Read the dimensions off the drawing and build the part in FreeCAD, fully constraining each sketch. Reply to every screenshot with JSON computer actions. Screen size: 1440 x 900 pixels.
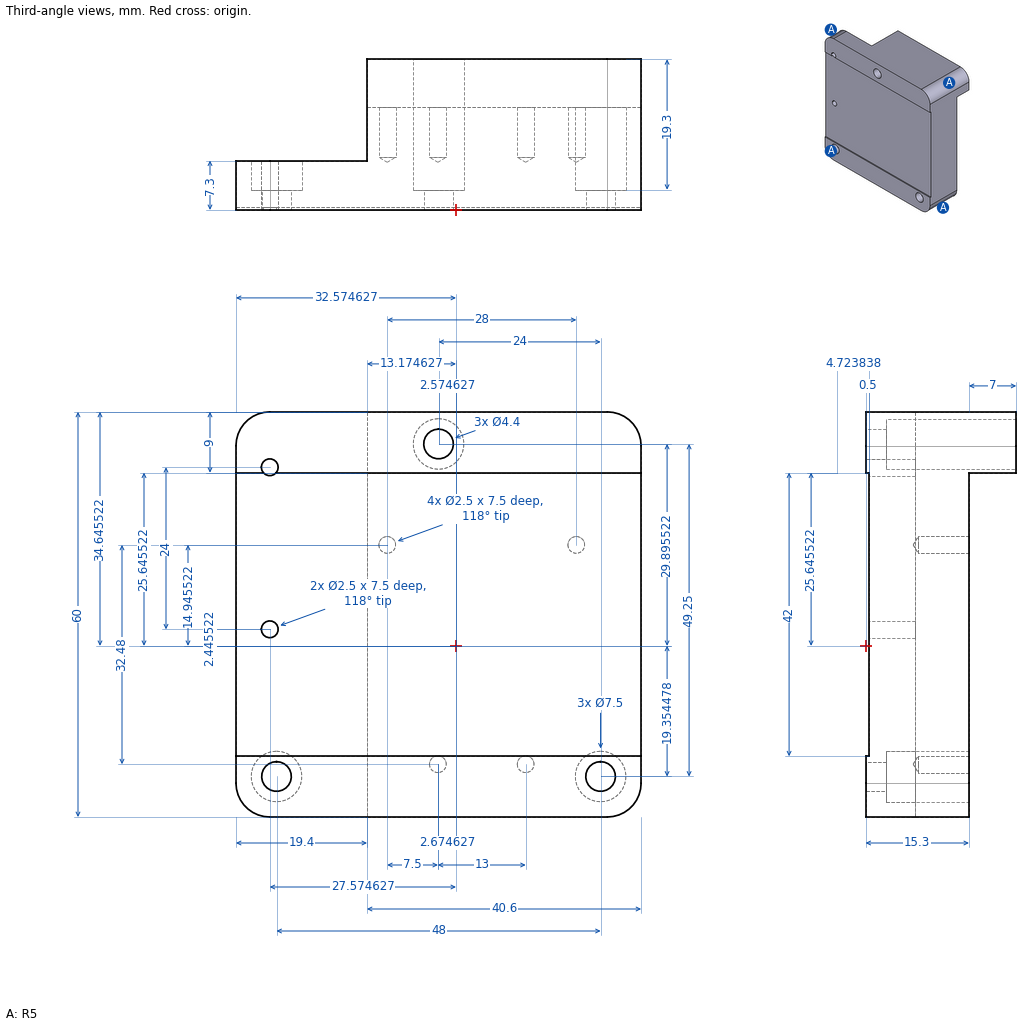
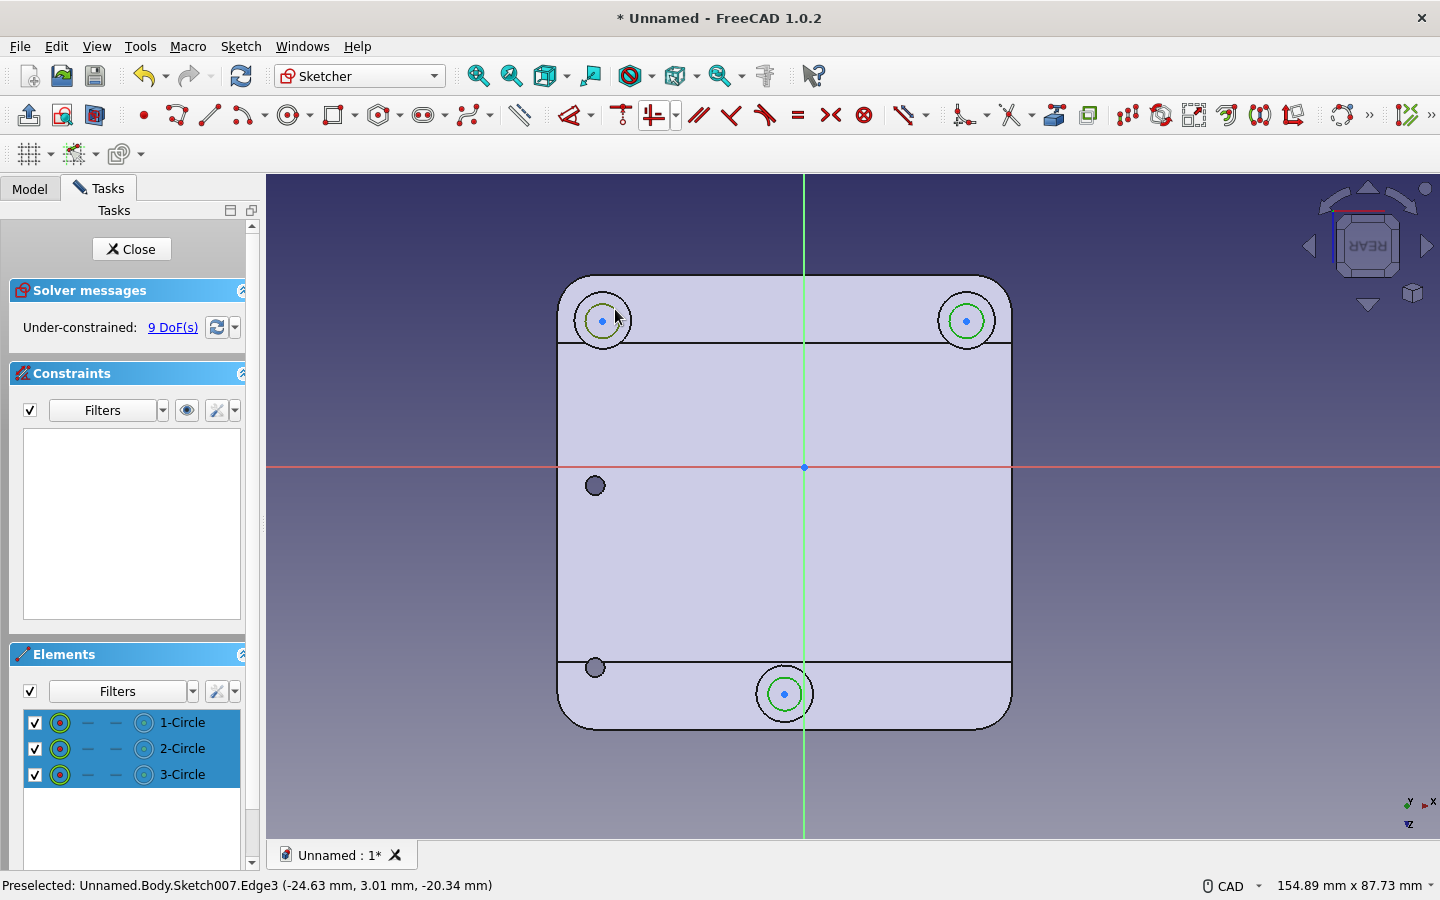
{"action": "key", "text": "e"}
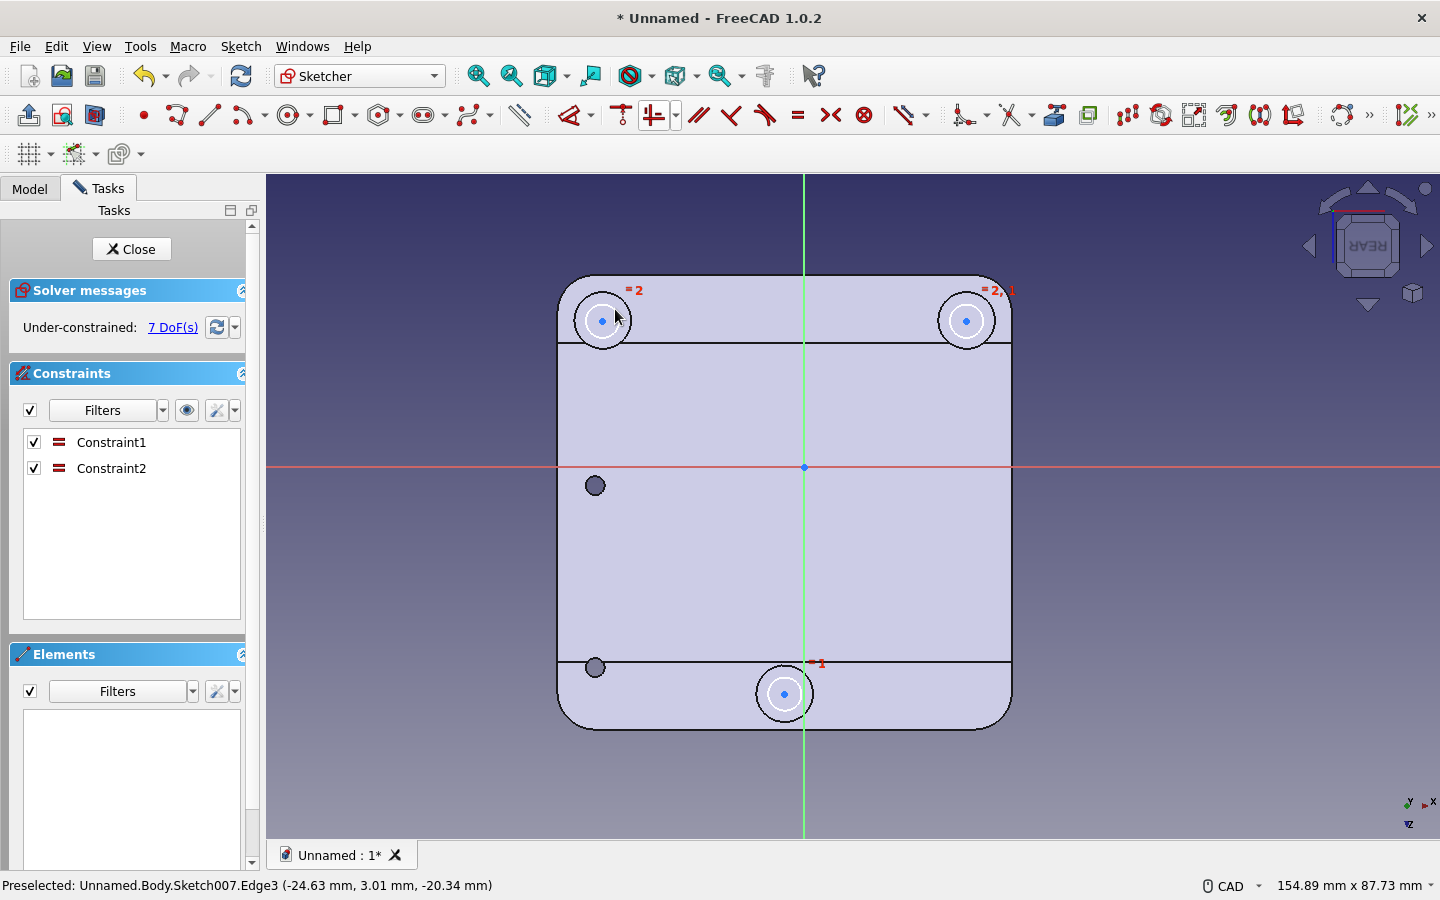
{"action": "left_click", "coordinate": [967, 321]}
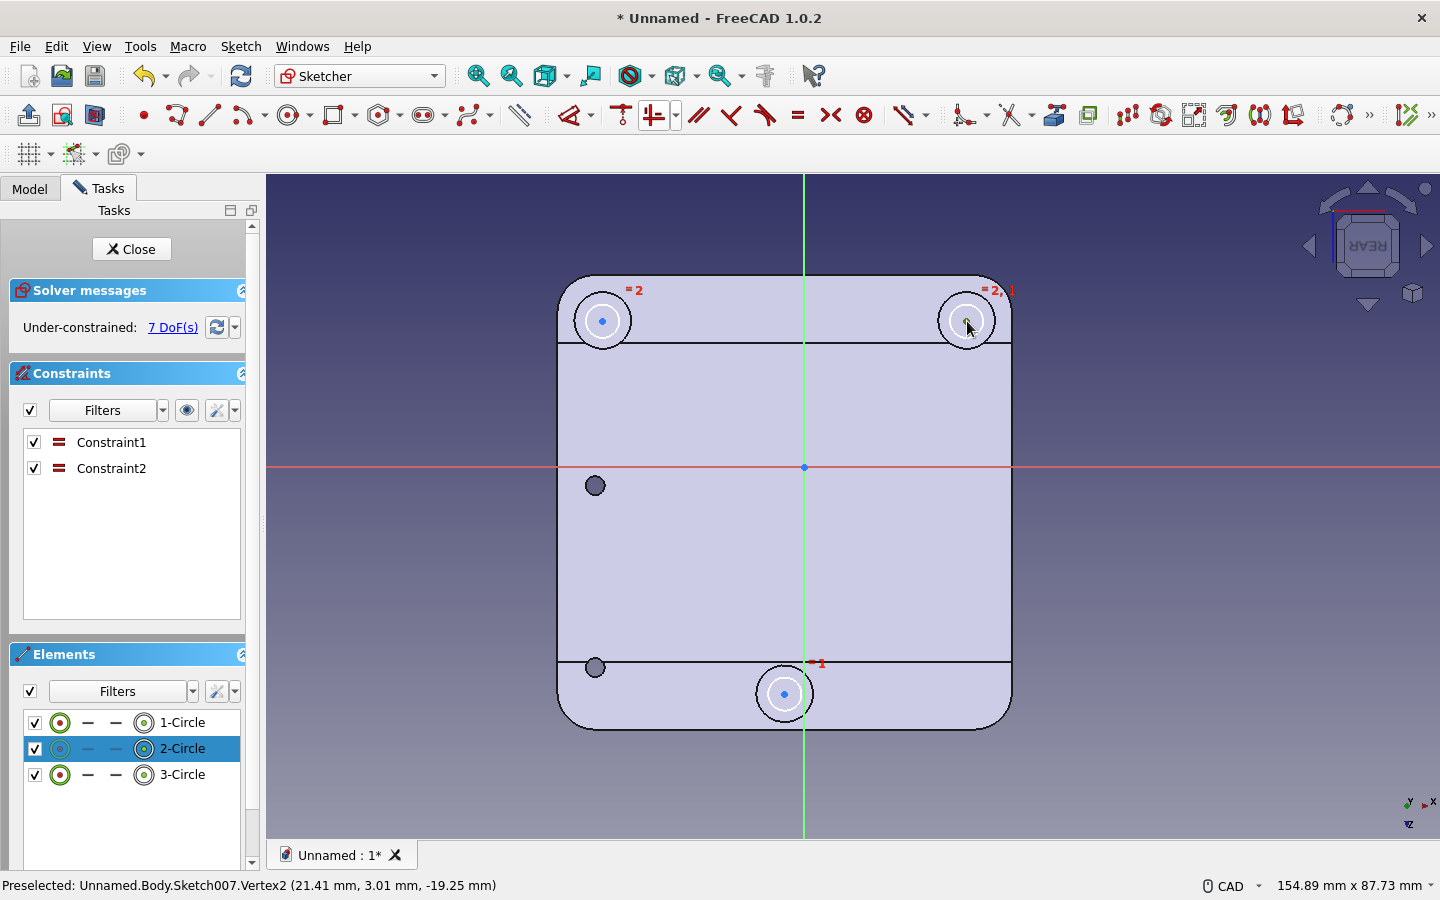
{"action": "left_click", "coordinate": [603, 321]}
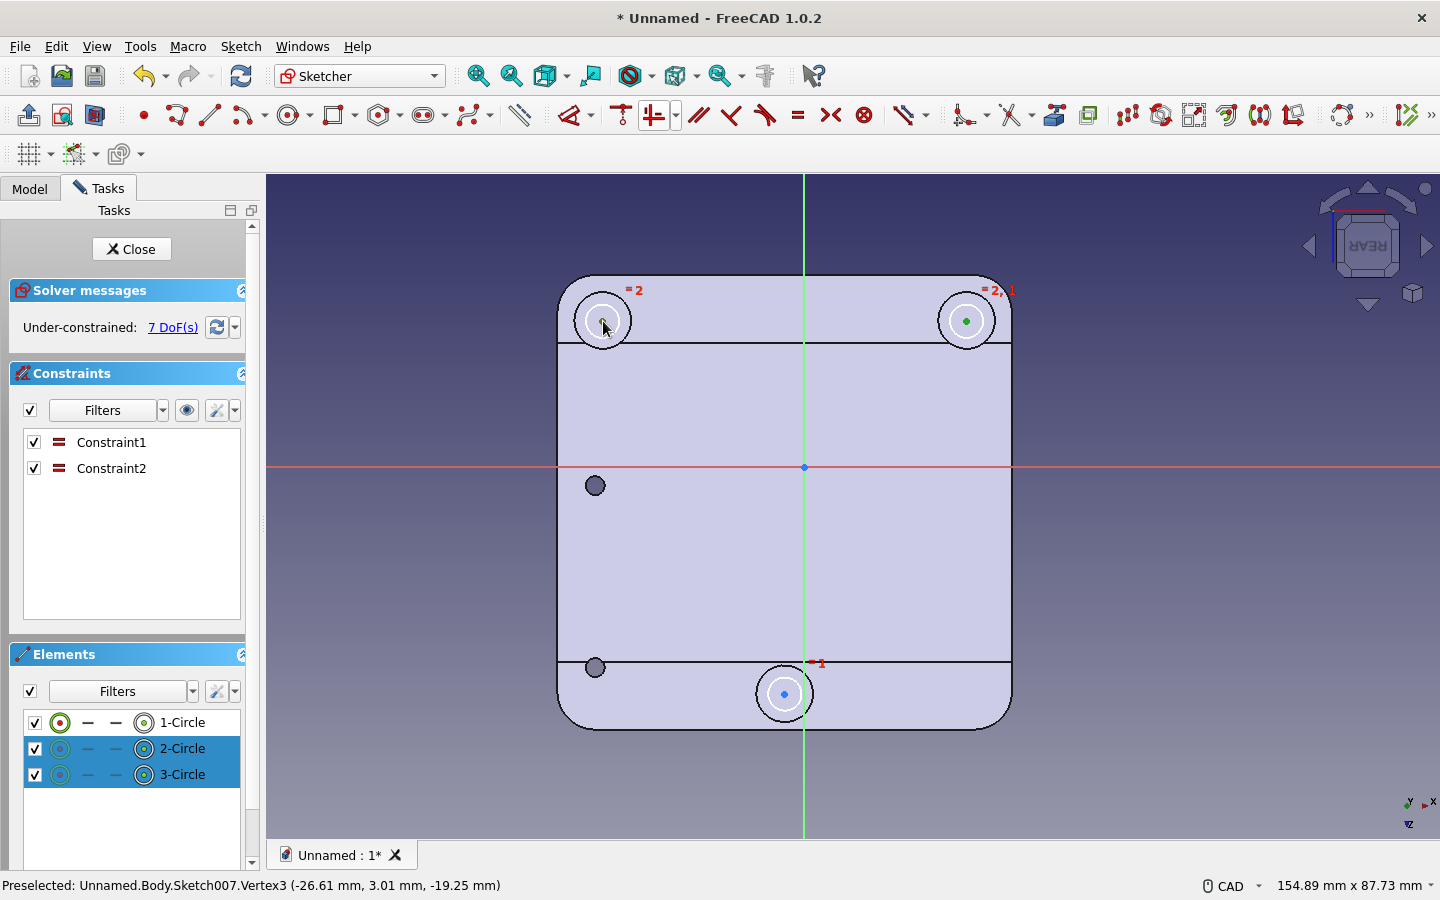
{"action": "key", "text": "h"}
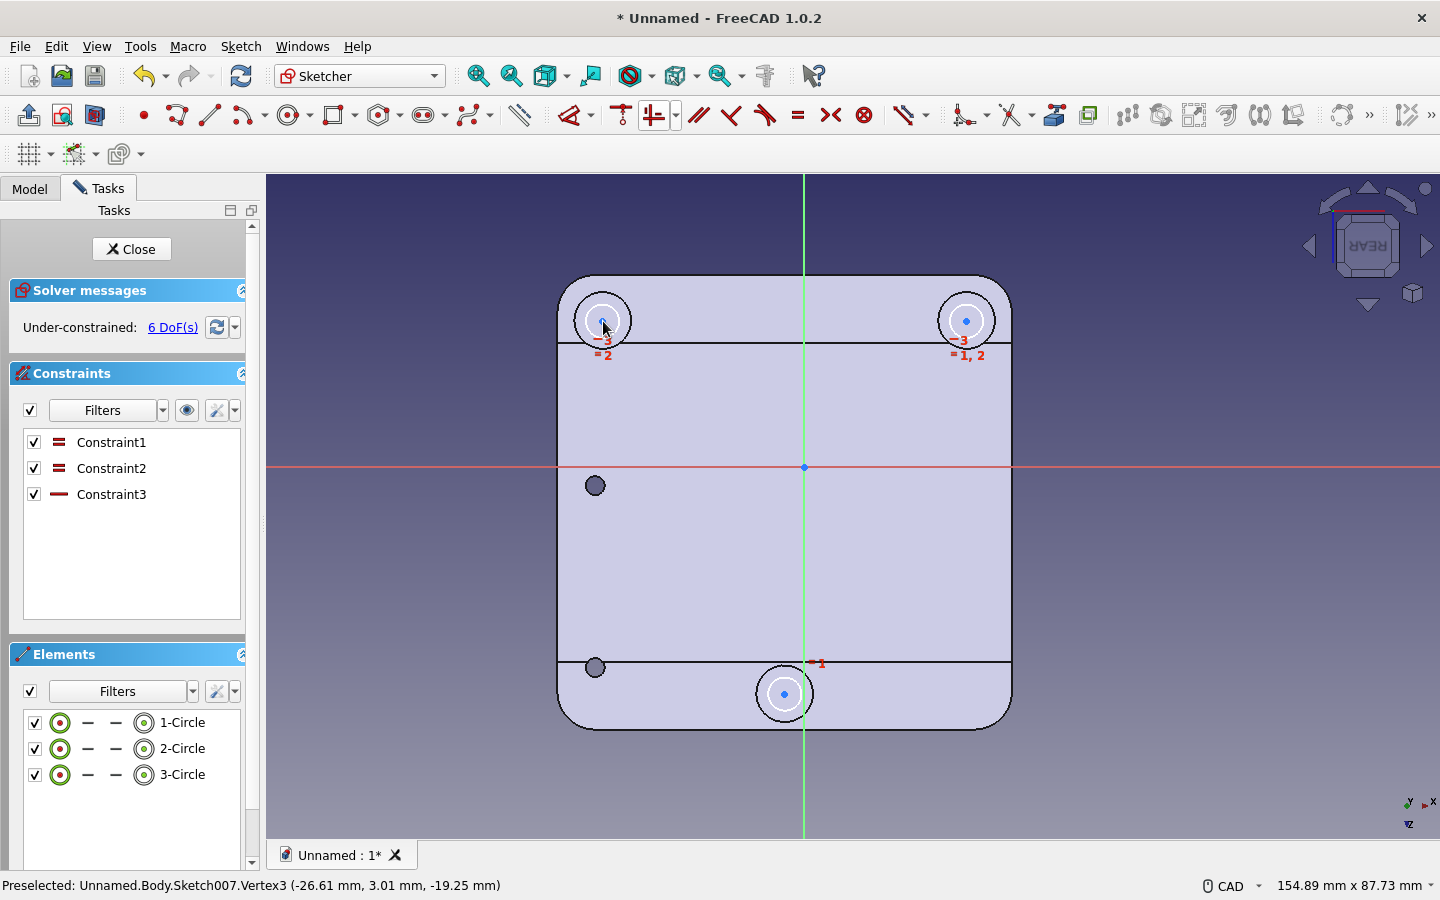
{"action": "key", "text": "d"}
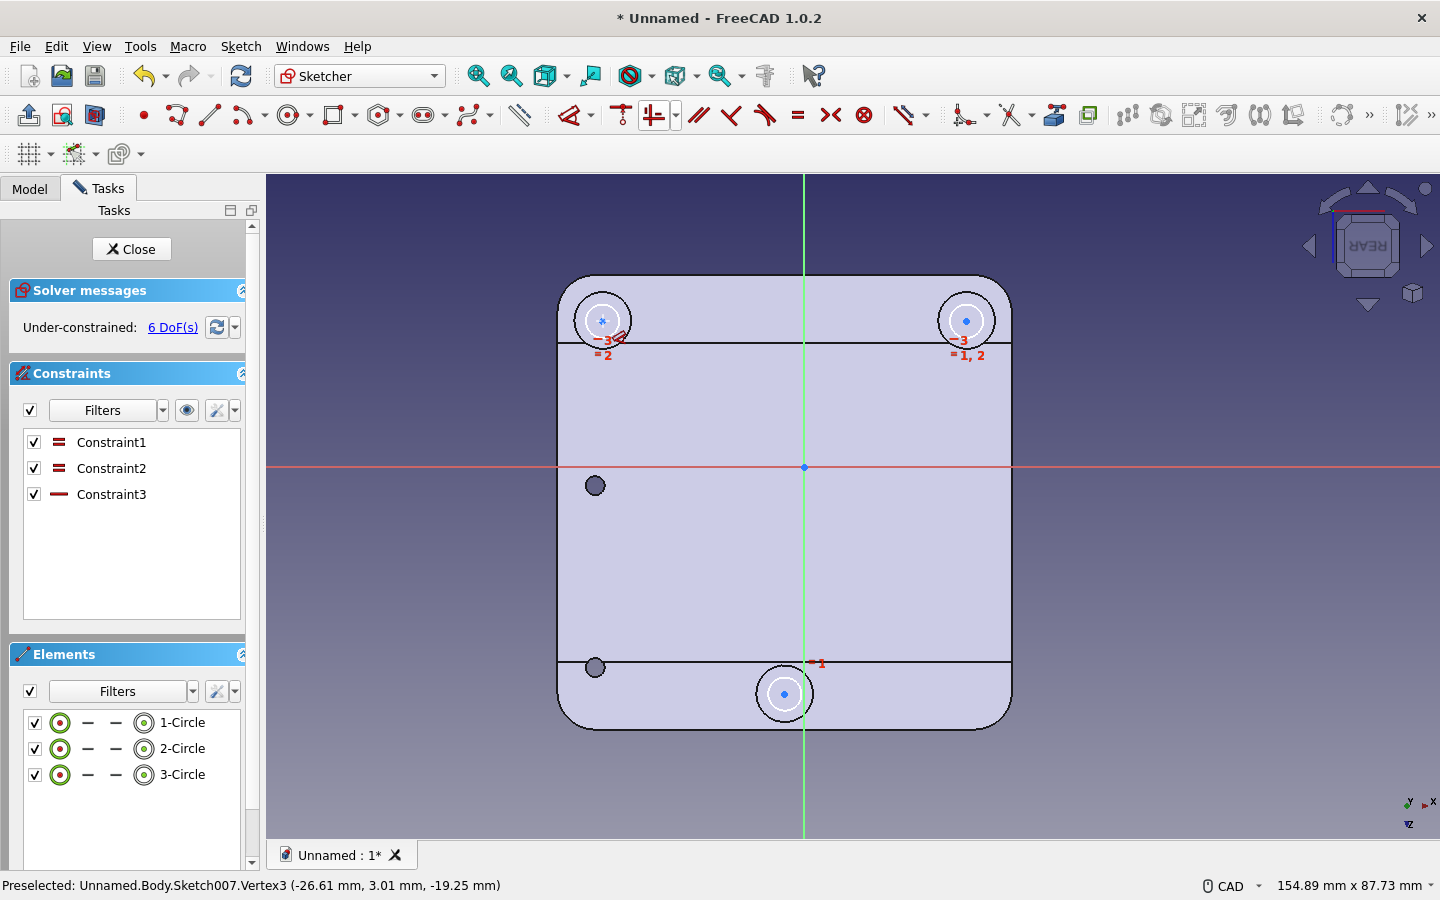
{"action": "left_click", "coordinate": [773, 682]}
{"action": "left_click", "coordinate": [751, 659]}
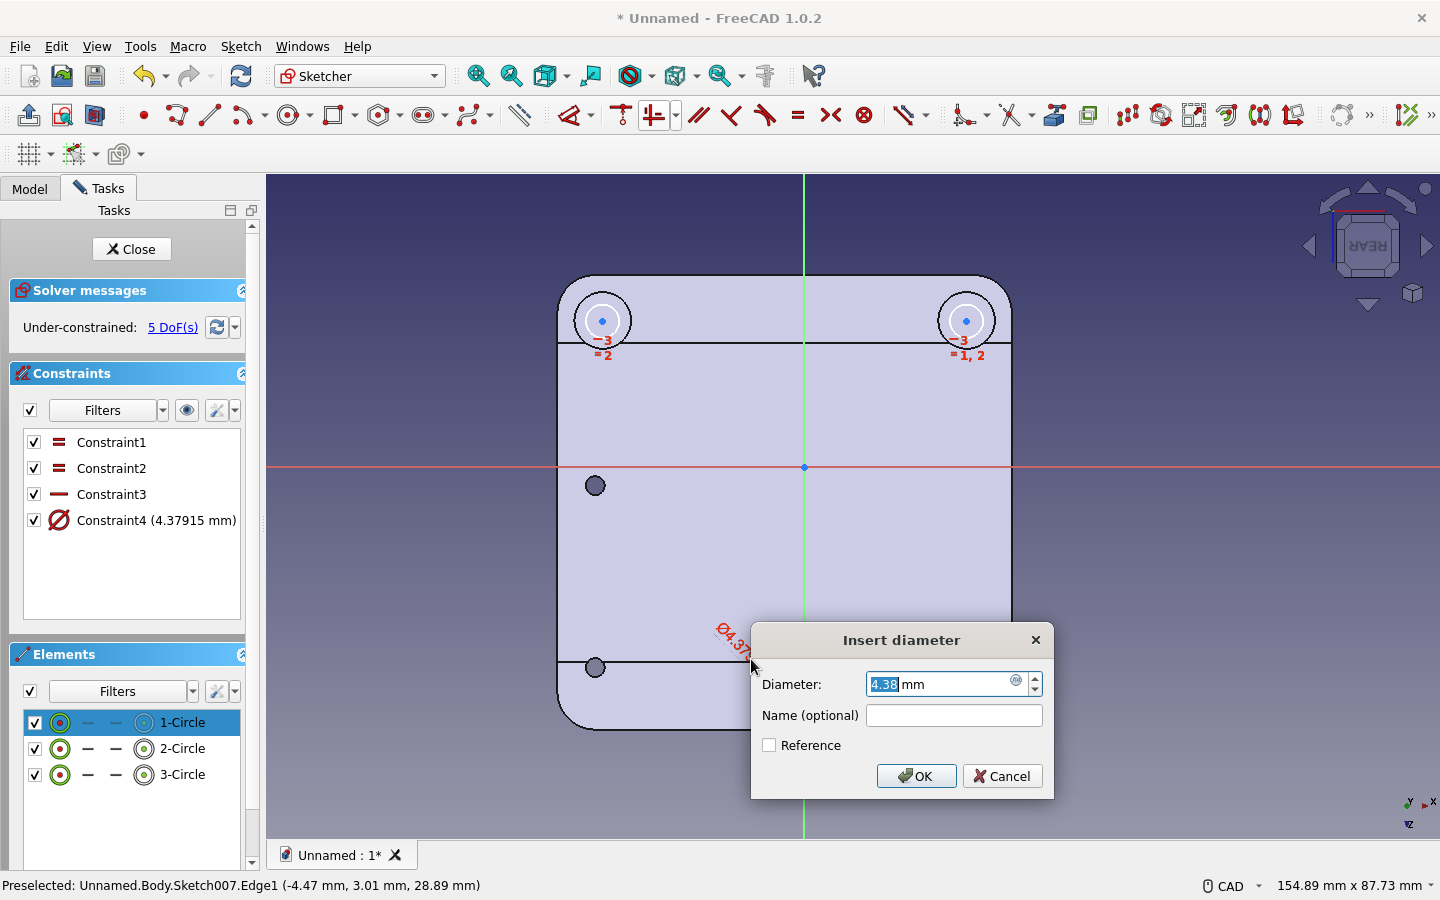
{"action": "type", "text": "4.4"}
{"action": "key", "text": "Return"}